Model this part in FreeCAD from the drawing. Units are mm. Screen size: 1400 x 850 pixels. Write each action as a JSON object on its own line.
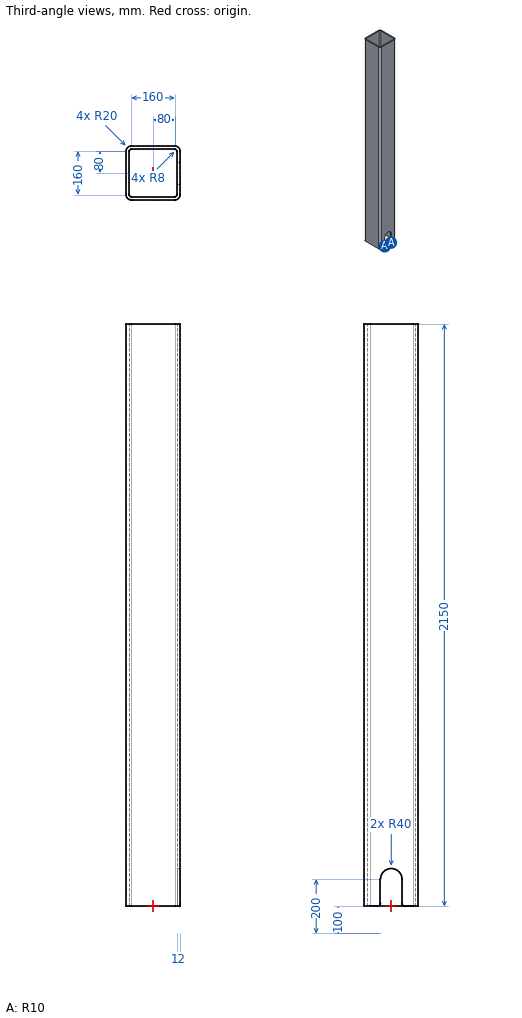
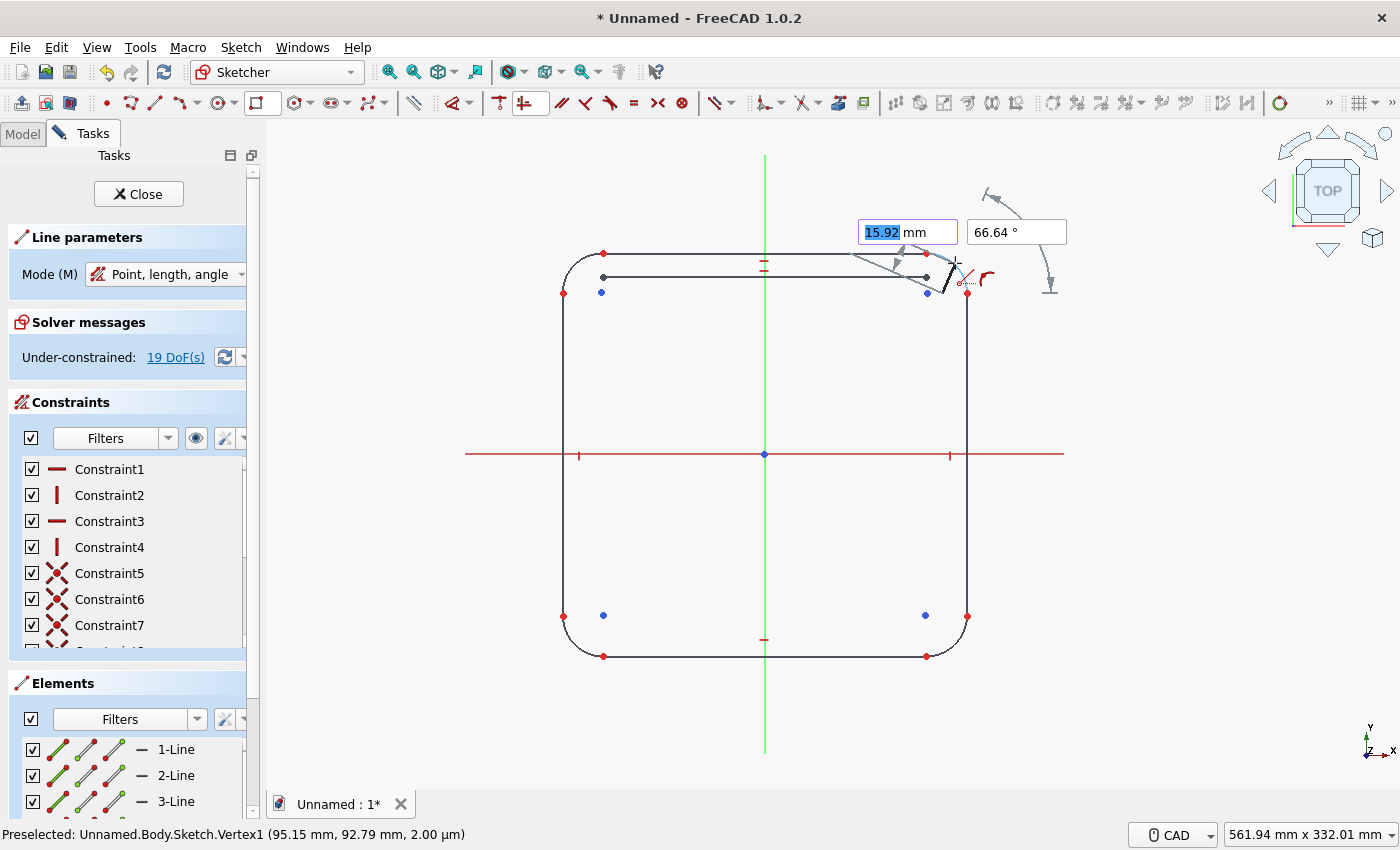
{"action": "left_click", "coordinate": [942, 615]}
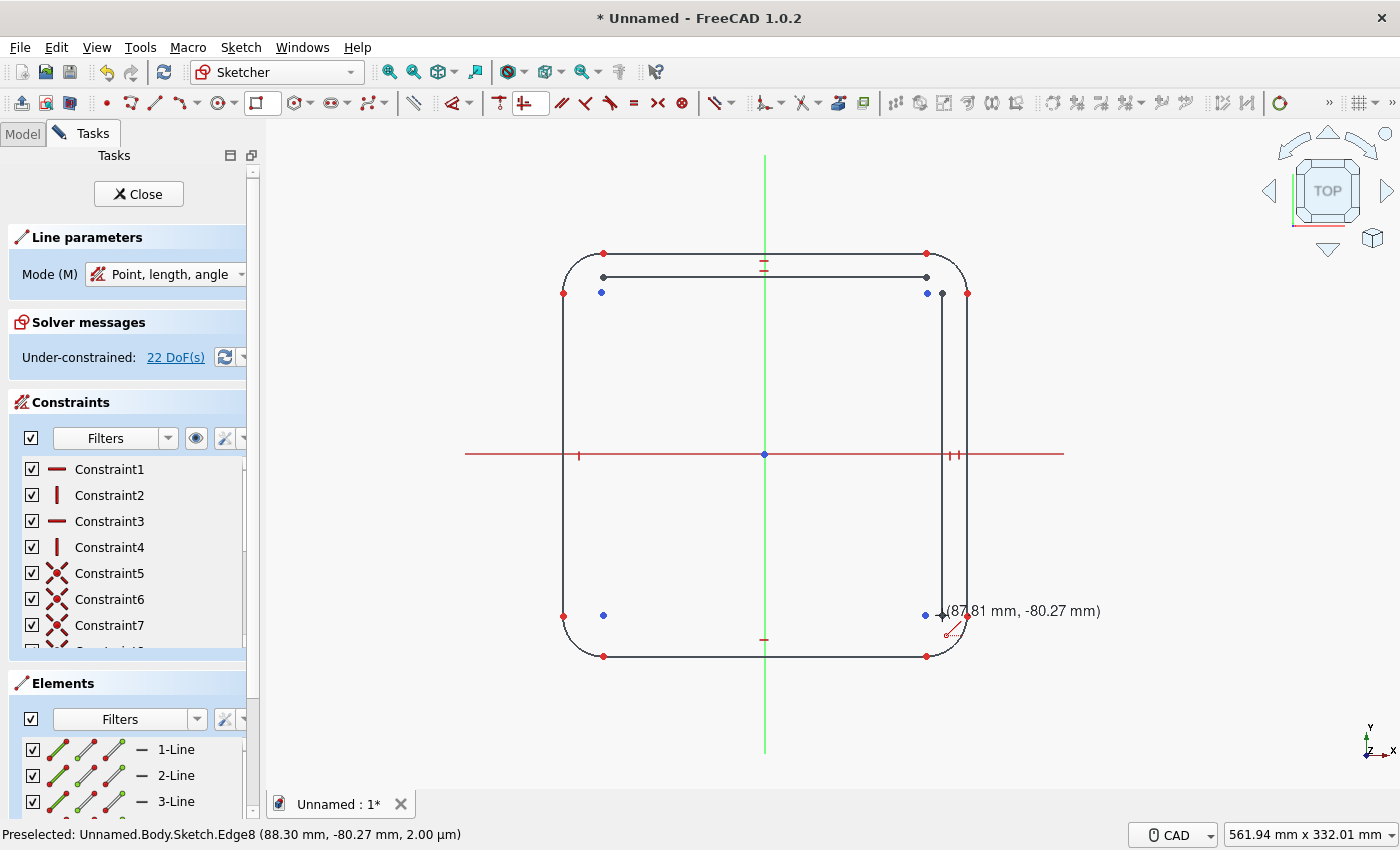
{"action": "left_click", "coordinate": [926, 632]}
{"action": "left_click", "coordinate": [603, 632]}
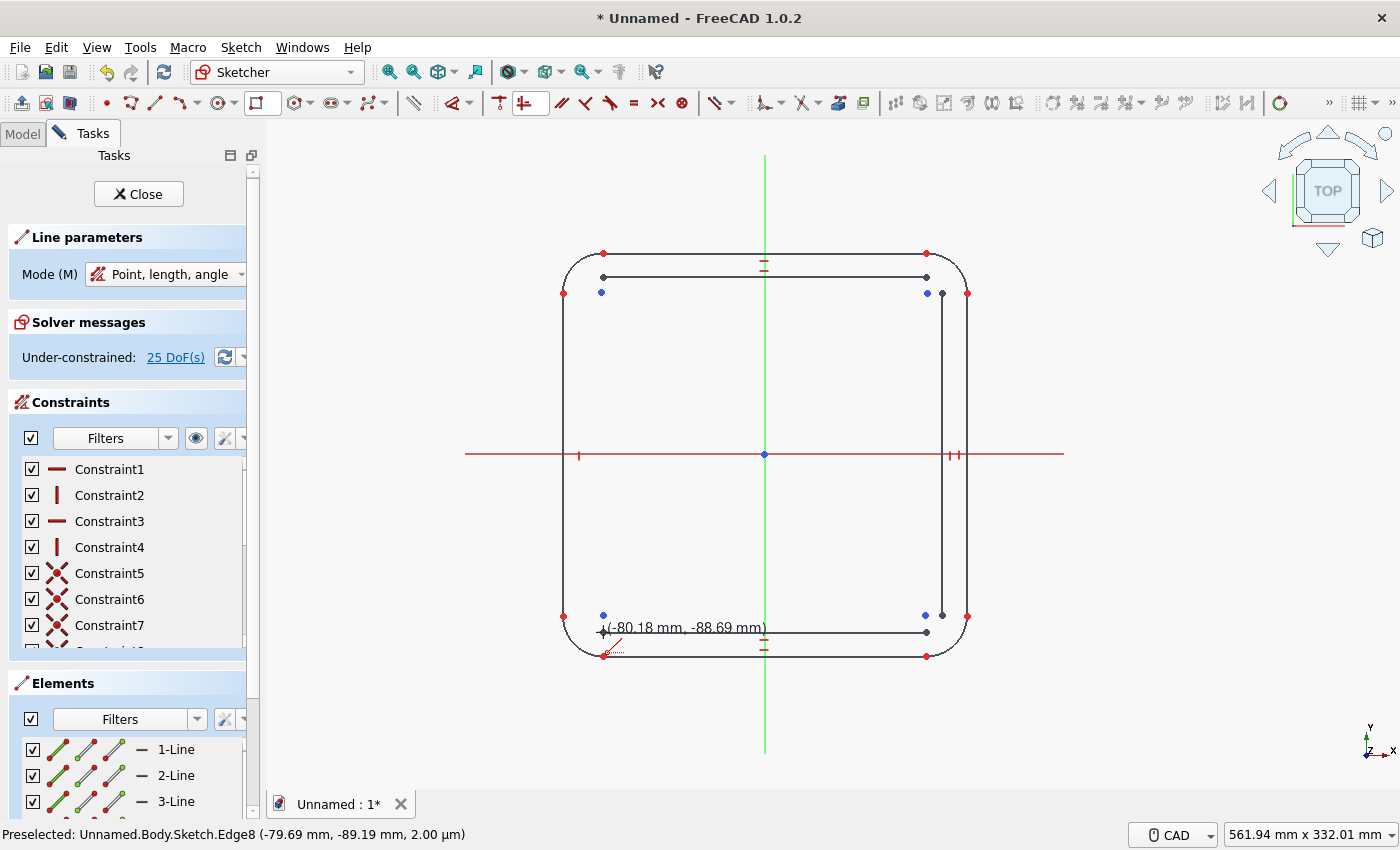
{"action": "left_click", "coordinate": [587, 615]}
{"action": "left_click", "coordinate": [587, 293]}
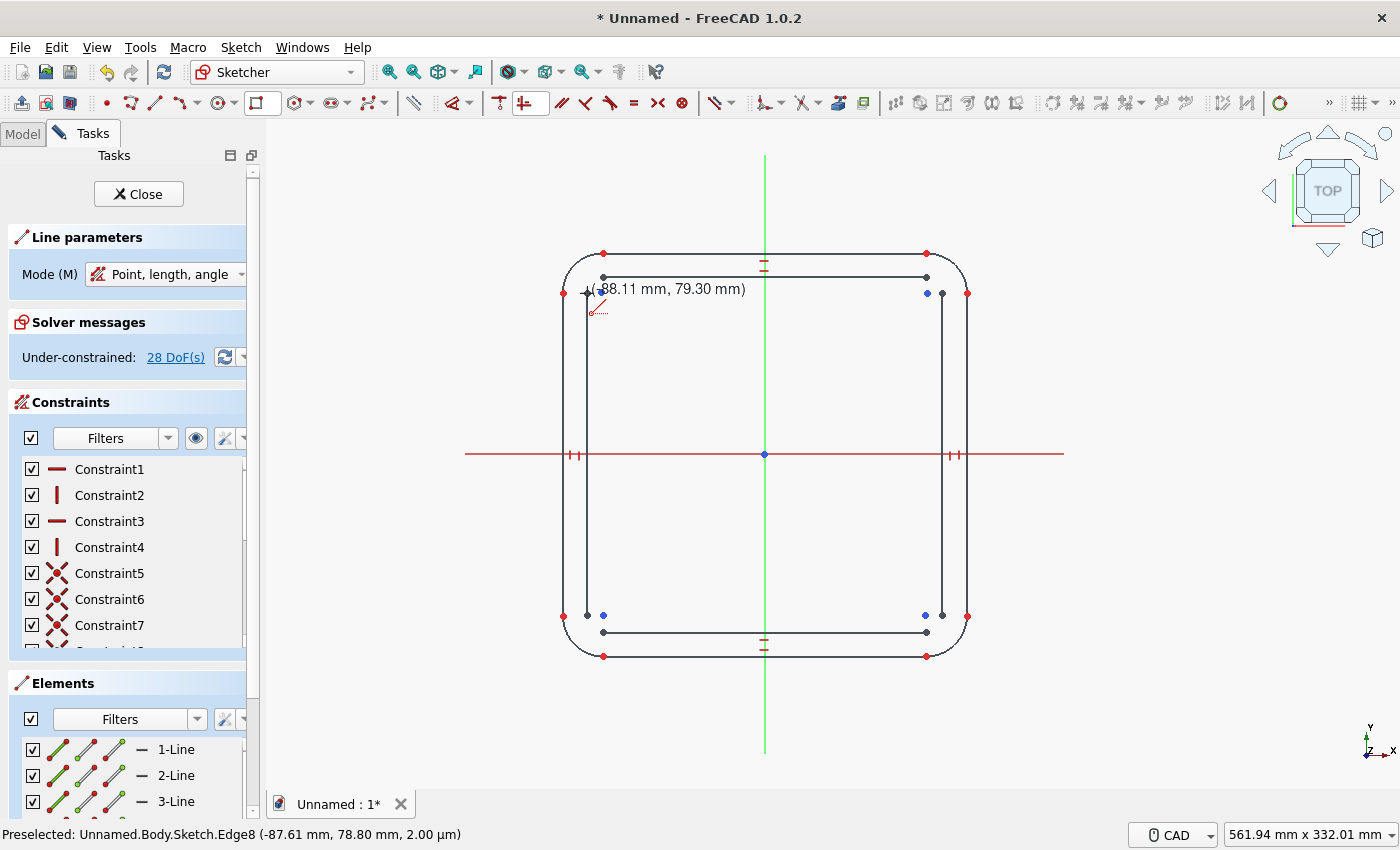
{"action": "left_click", "coordinate": [180, 104]}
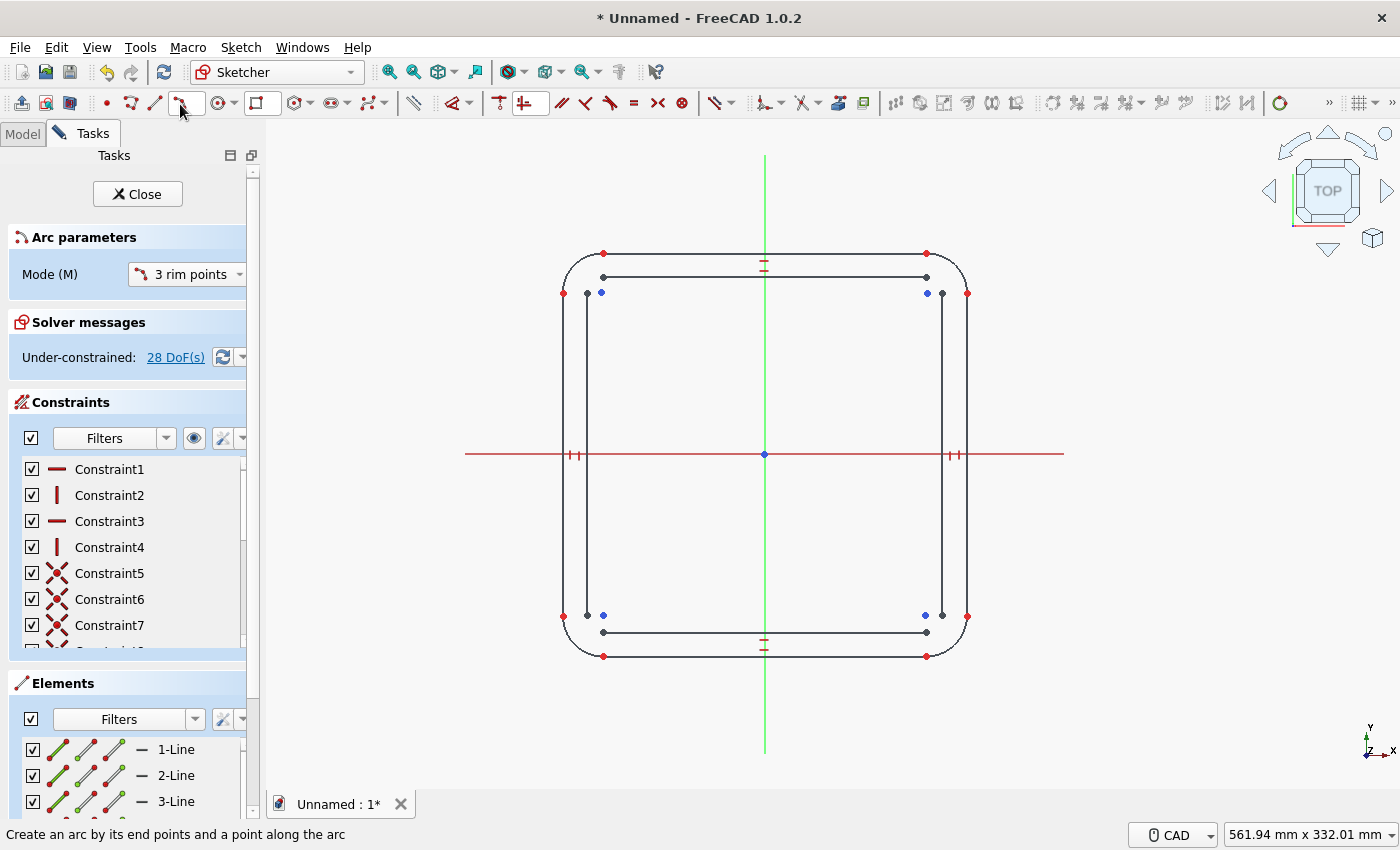
{"action": "left_click", "coordinate": [926, 277]}
{"action": "left_click", "coordinate": [942, 293]}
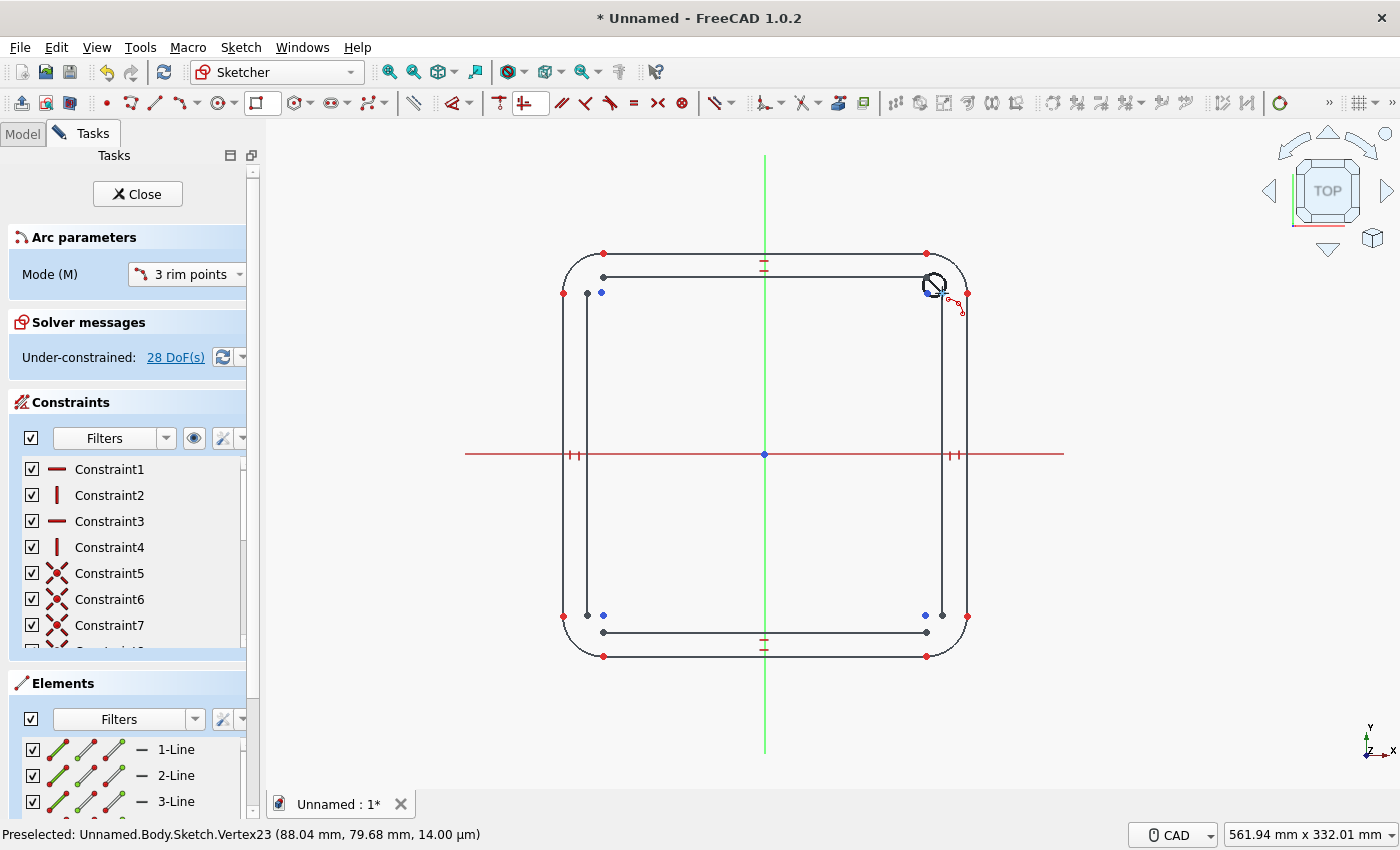
{"action": "scroll", "coordinate": [938, 281], "scroll_direction": "up", "scroll_amount": 7}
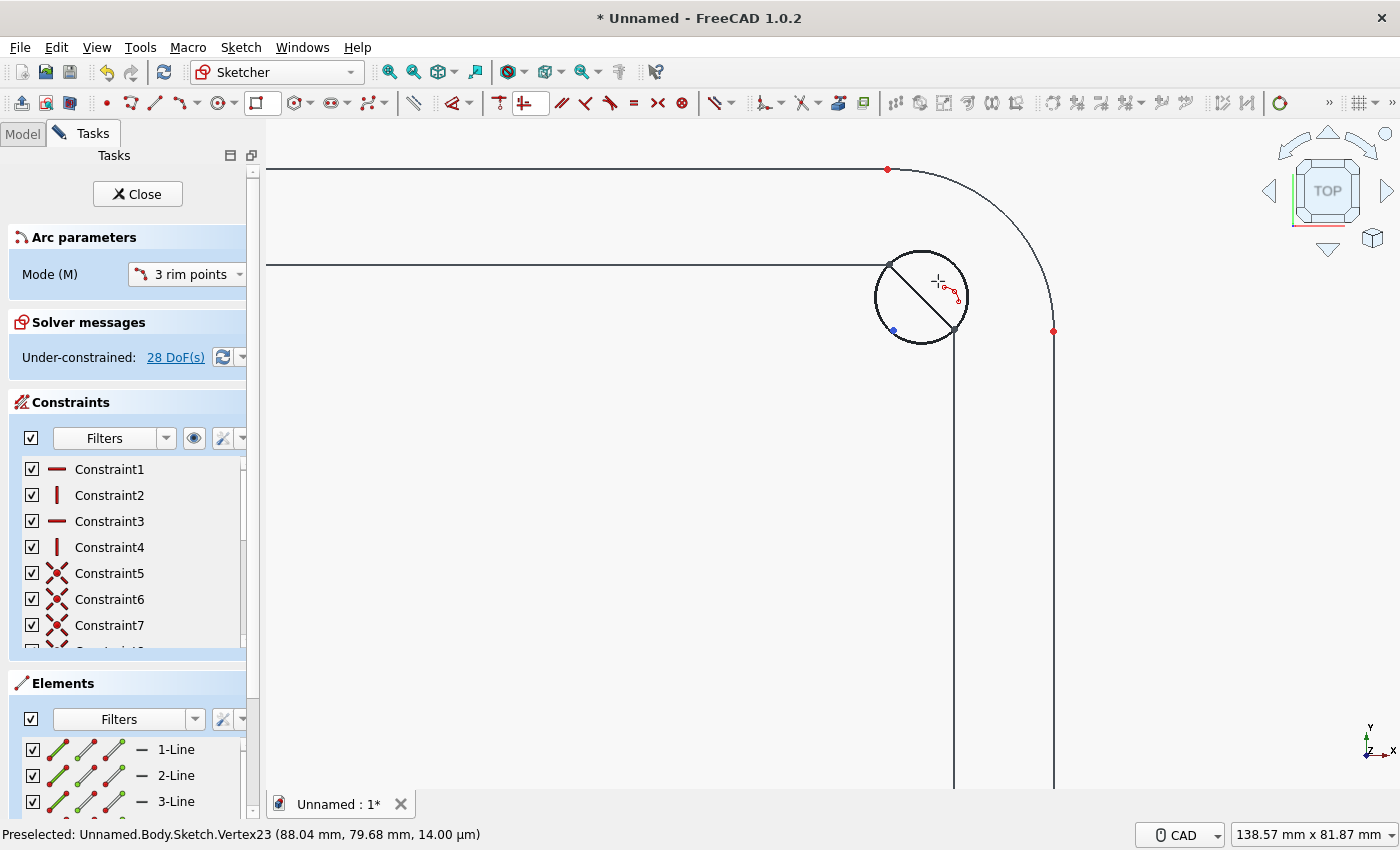
{"action": "left_click", "coordinate": [935, 281]}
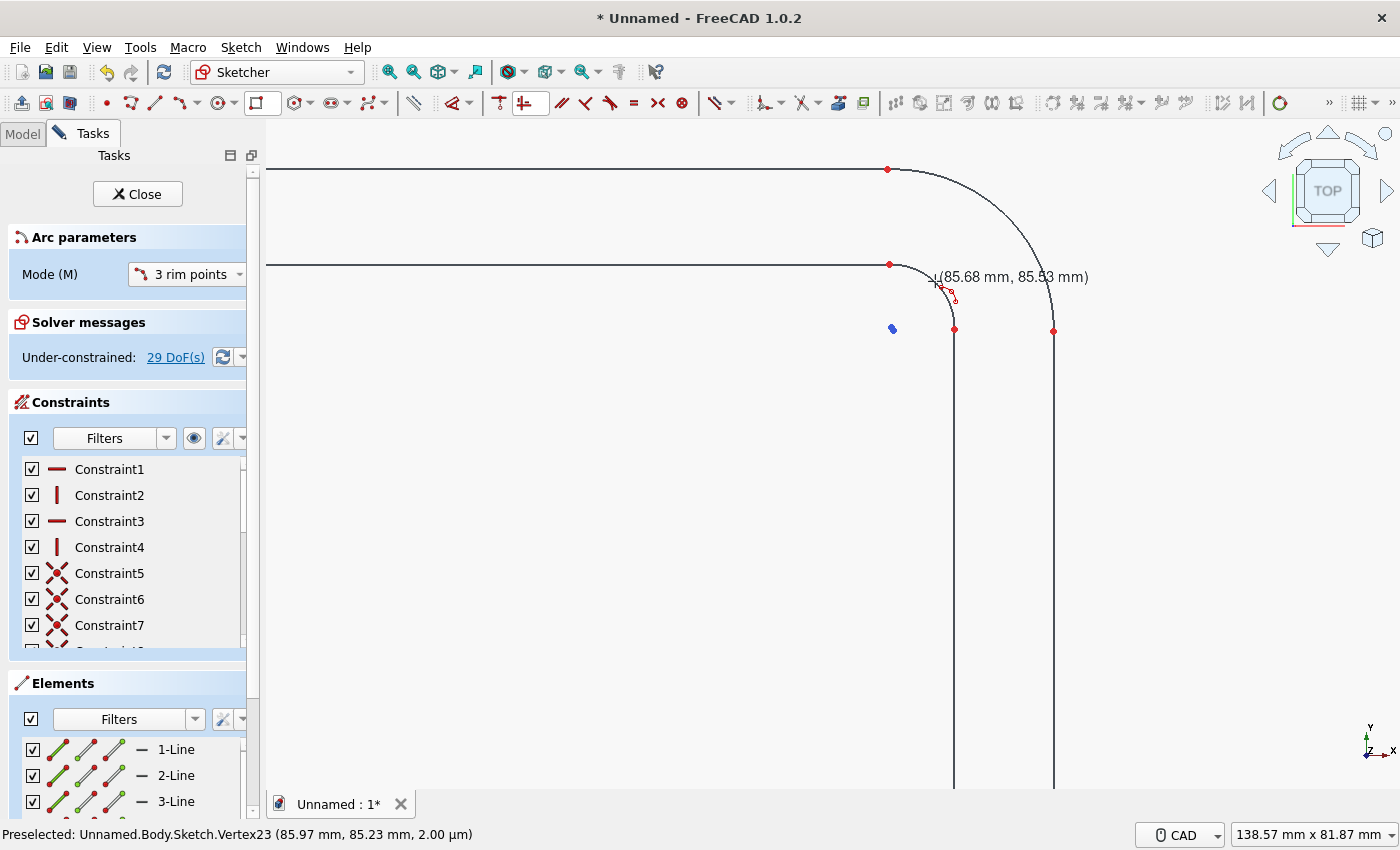
{"action": "scroll", "coordinate": [938, 281], "scroll_direction": "down", "scroll_amount": 7}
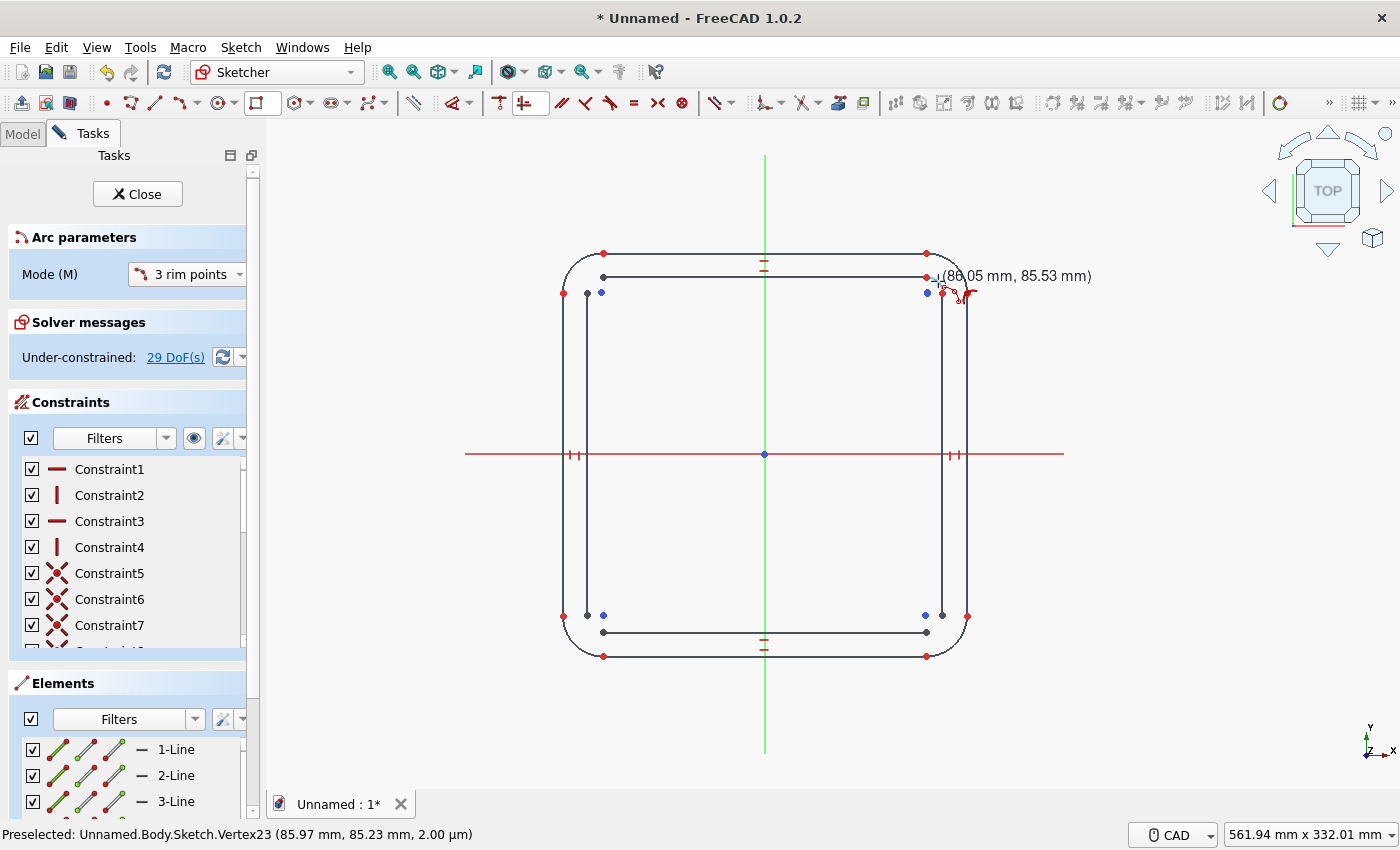
{"action": "left_click", "coordinate": [942, 616]}
{"action": "left_click", "coordinate": [926, 633]}